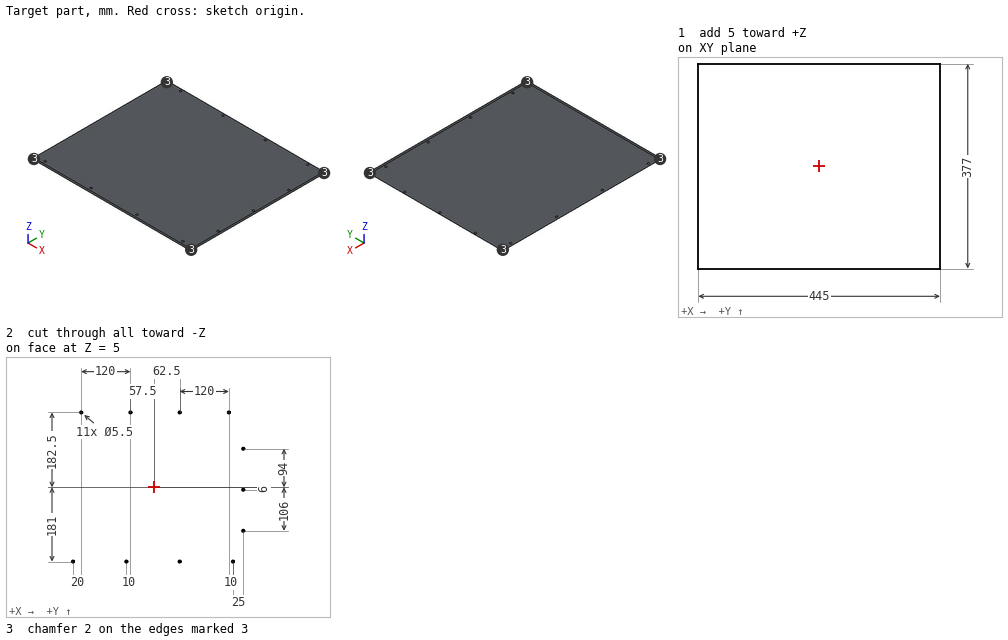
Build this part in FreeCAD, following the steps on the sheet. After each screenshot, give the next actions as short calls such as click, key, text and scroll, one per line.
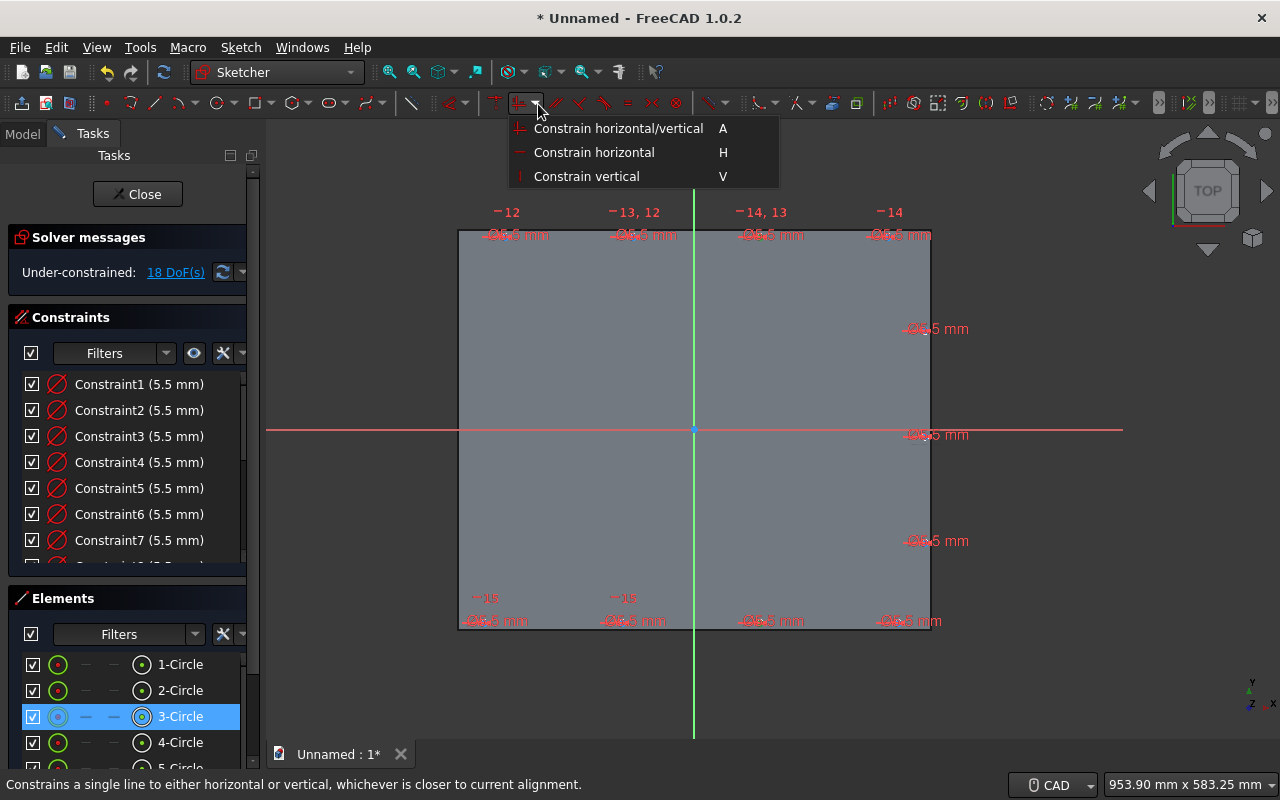
click(644, 176)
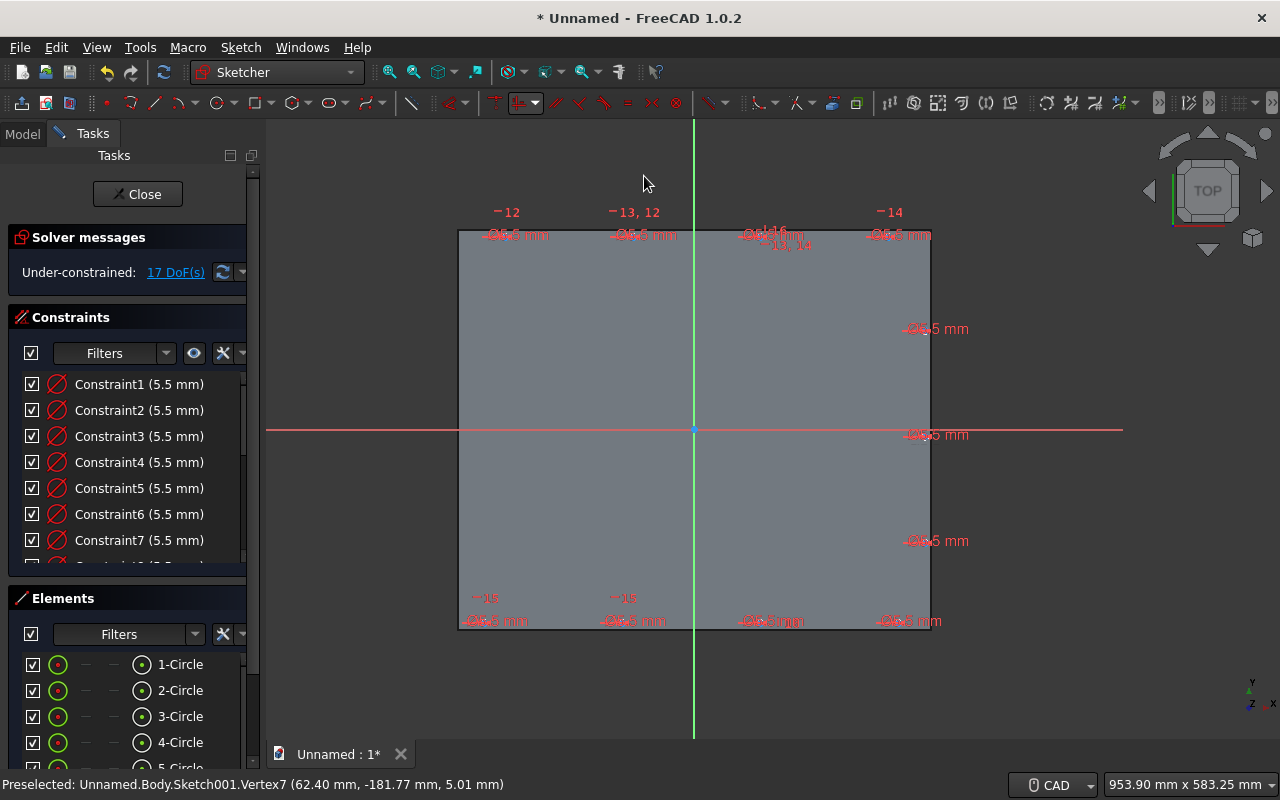
click(622, 623)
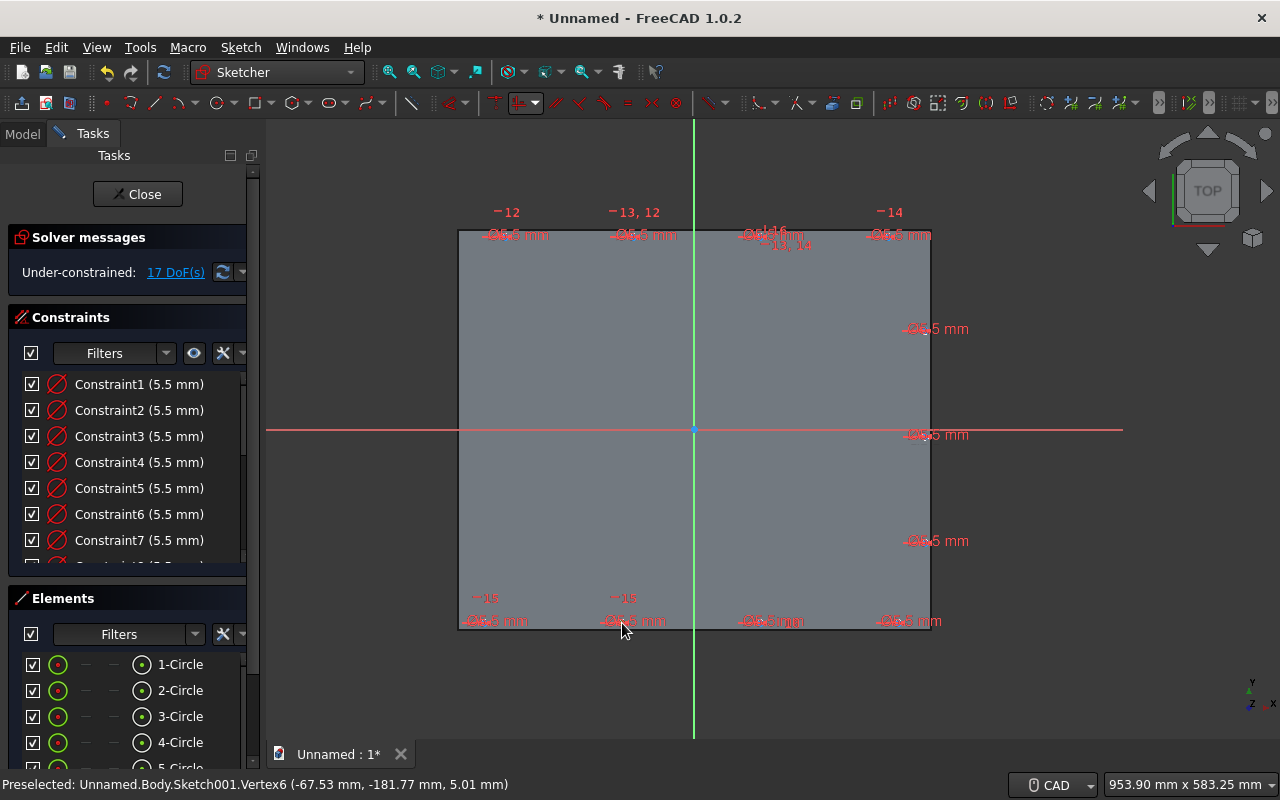
click(760, 623)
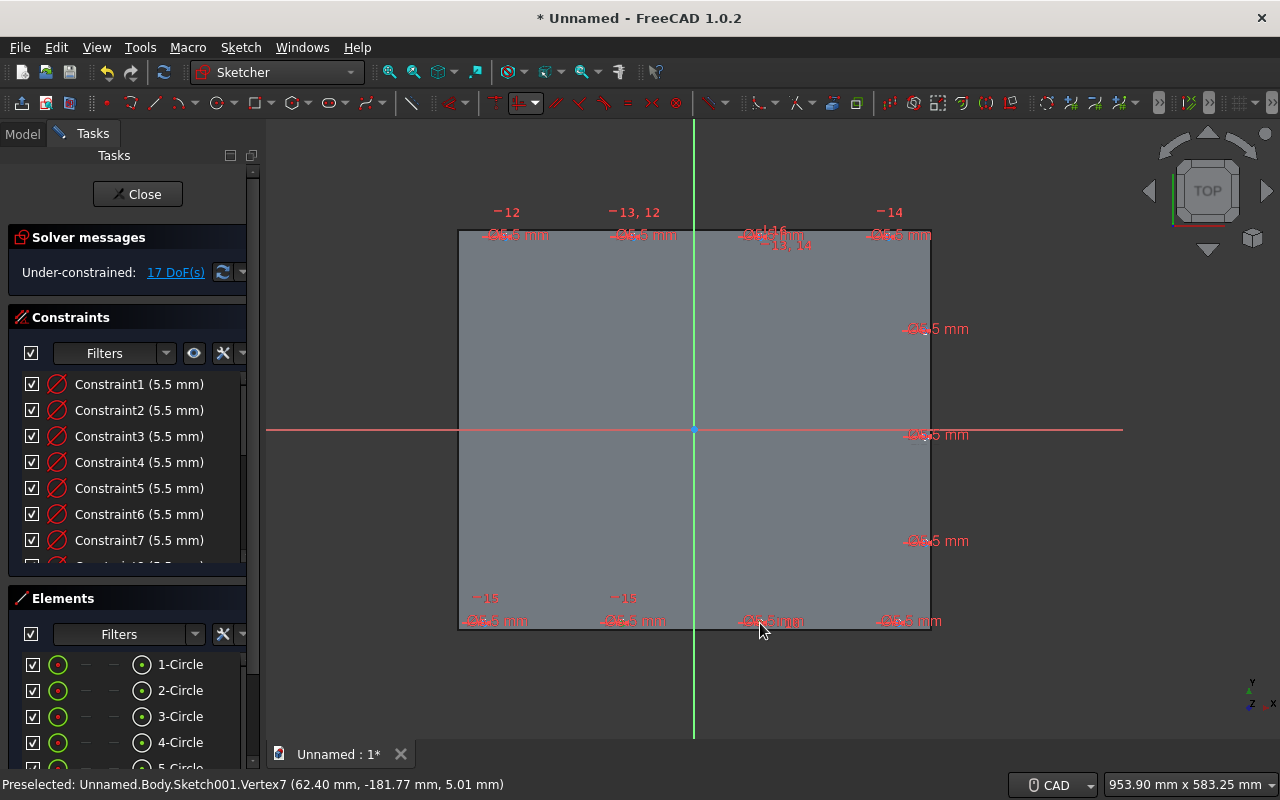
key(h)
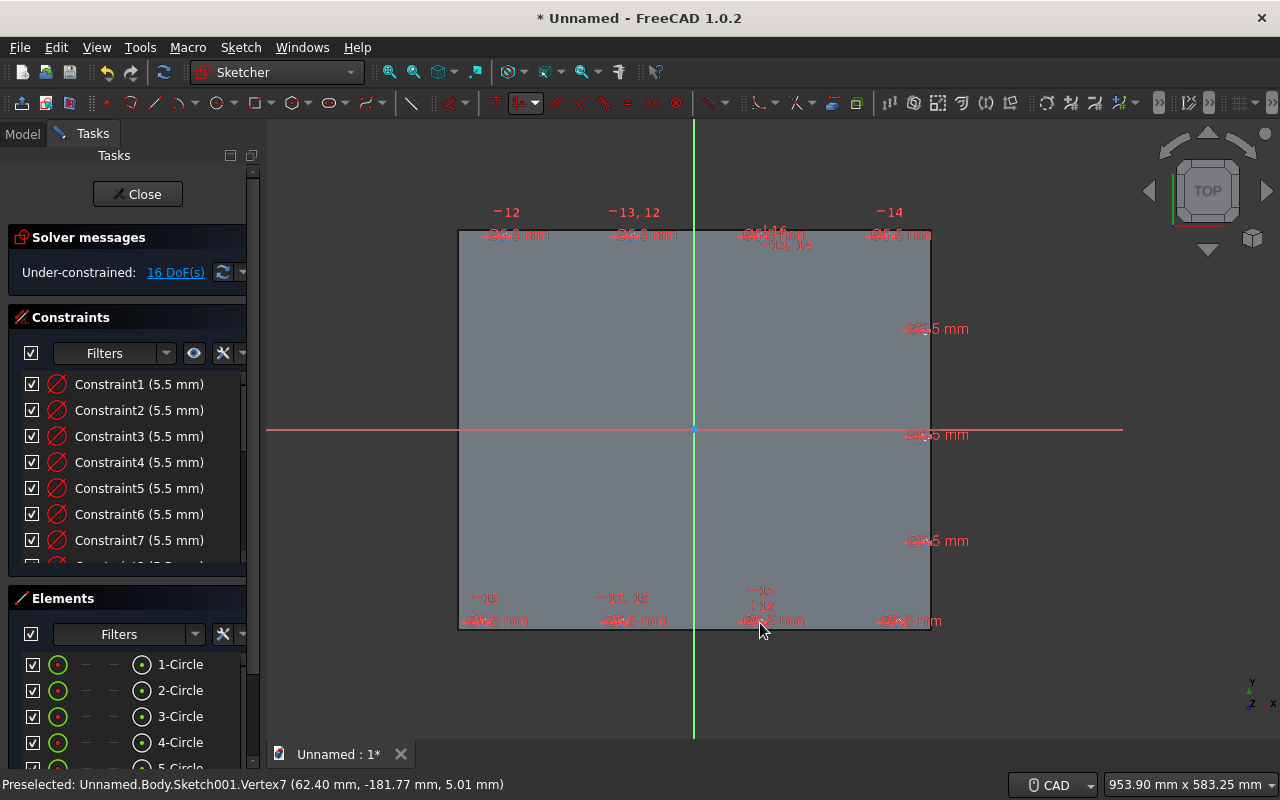
click(760, 623)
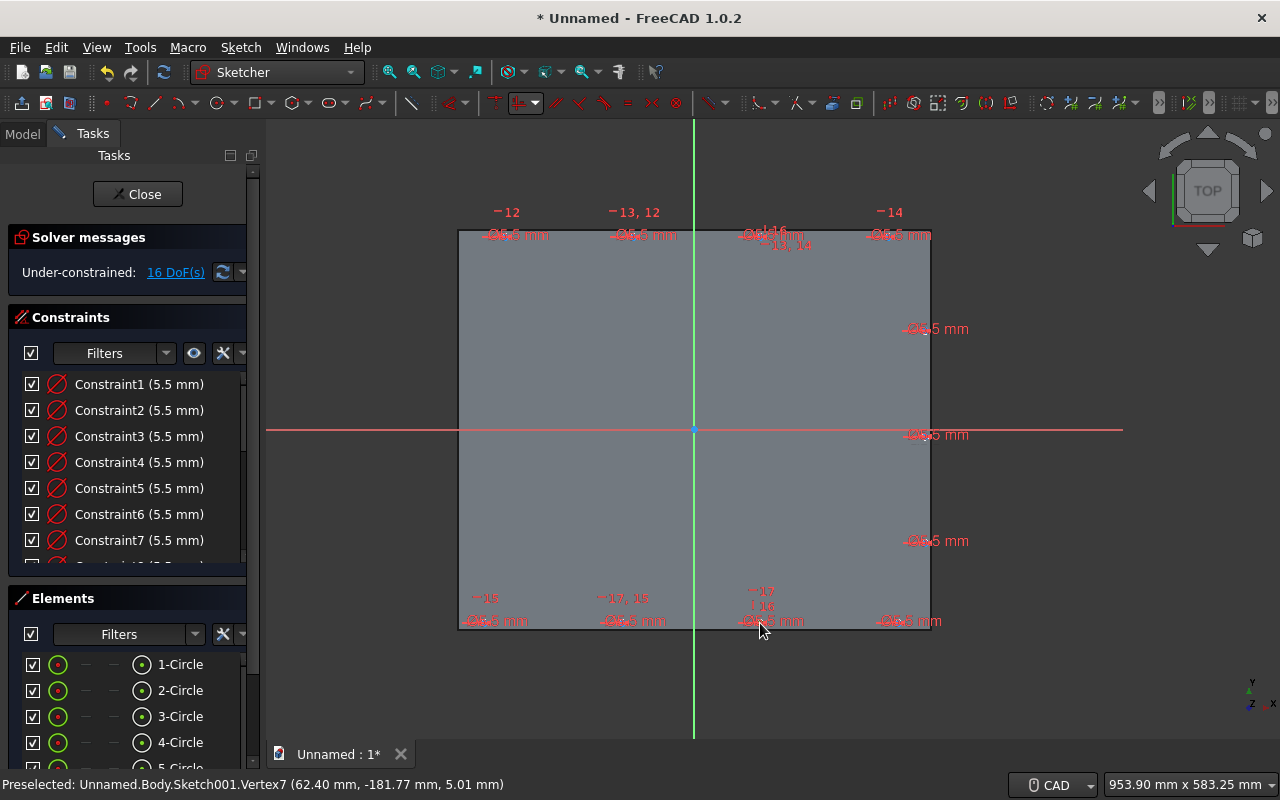
click(898, 623)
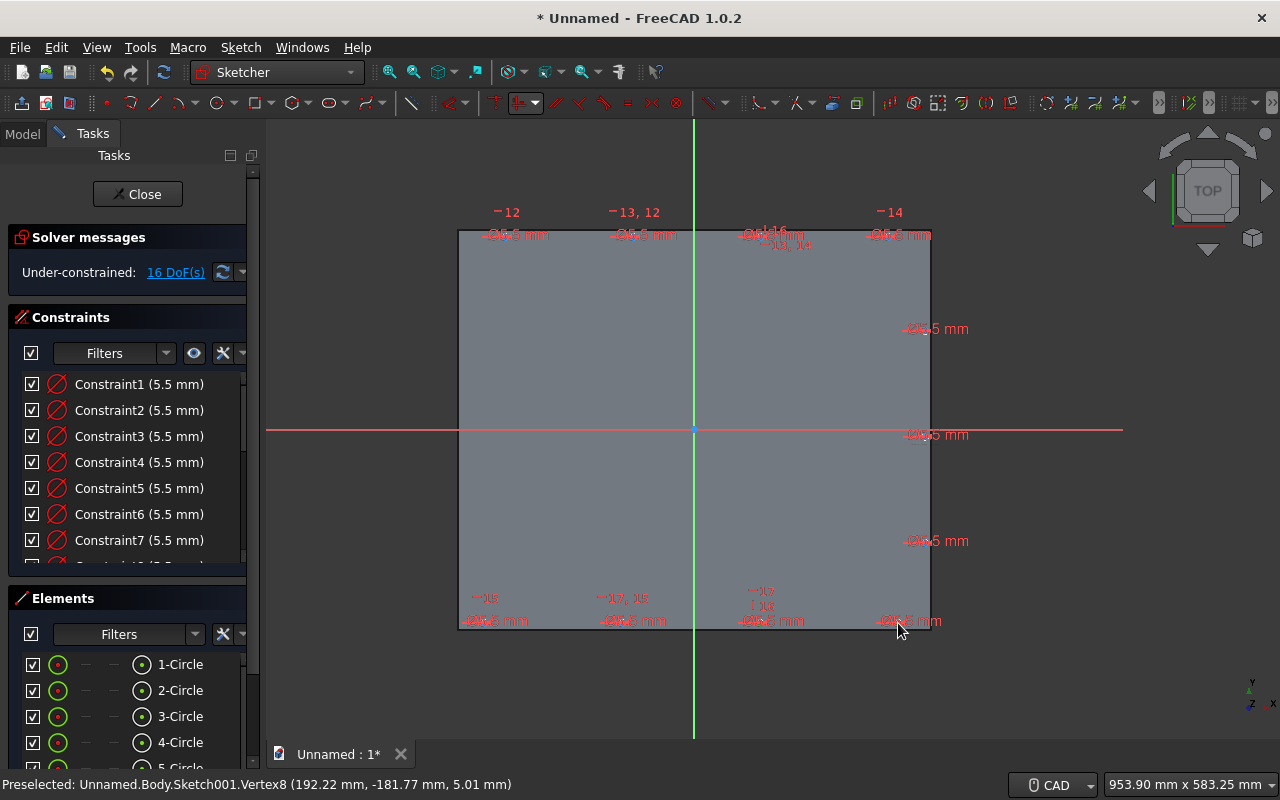
click(538, 104)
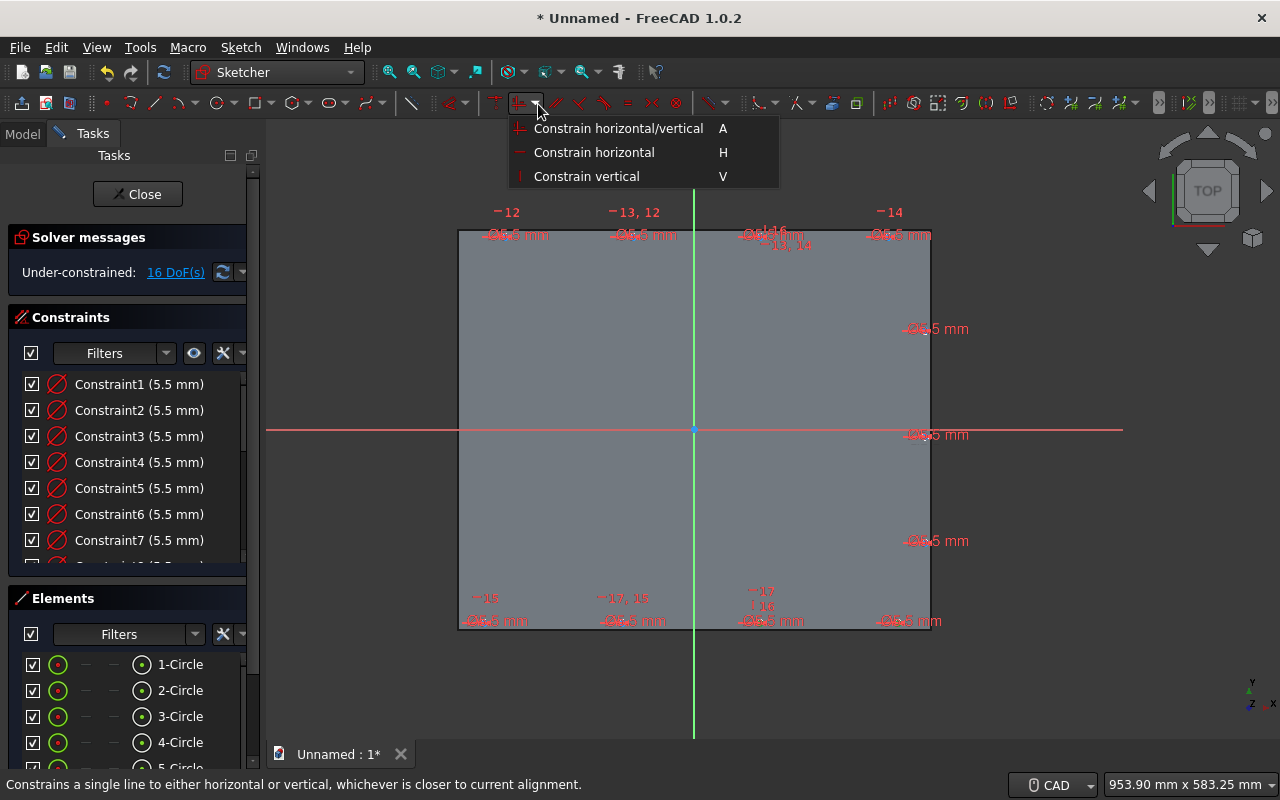
click(644, 152)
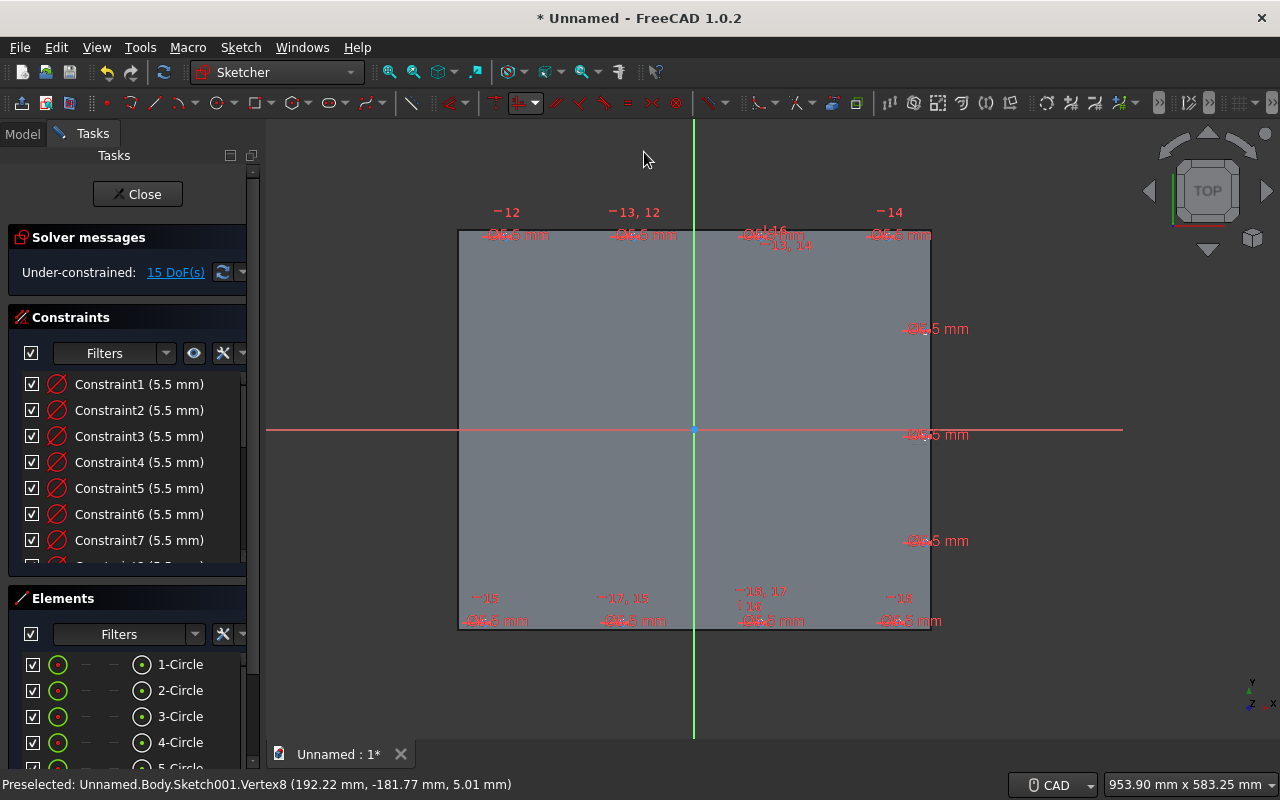
click(925, 543)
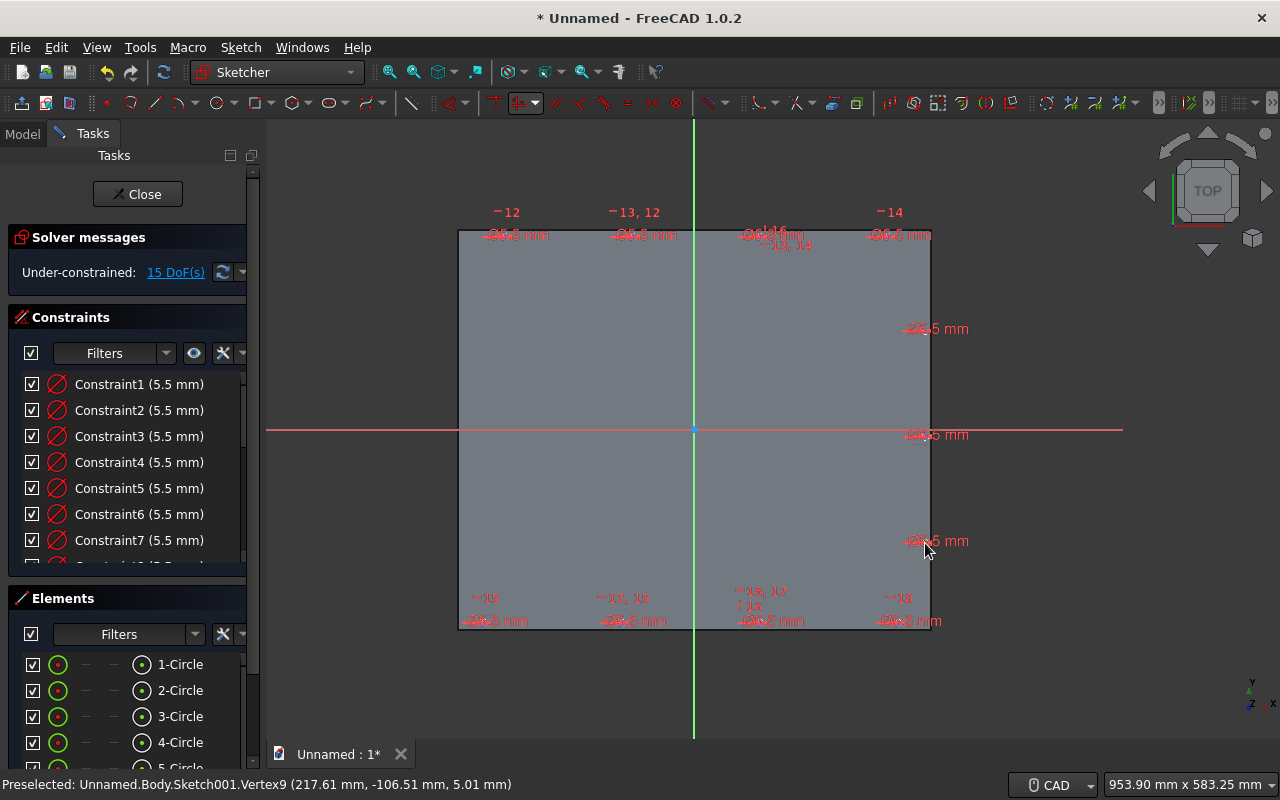
click(925, 437)